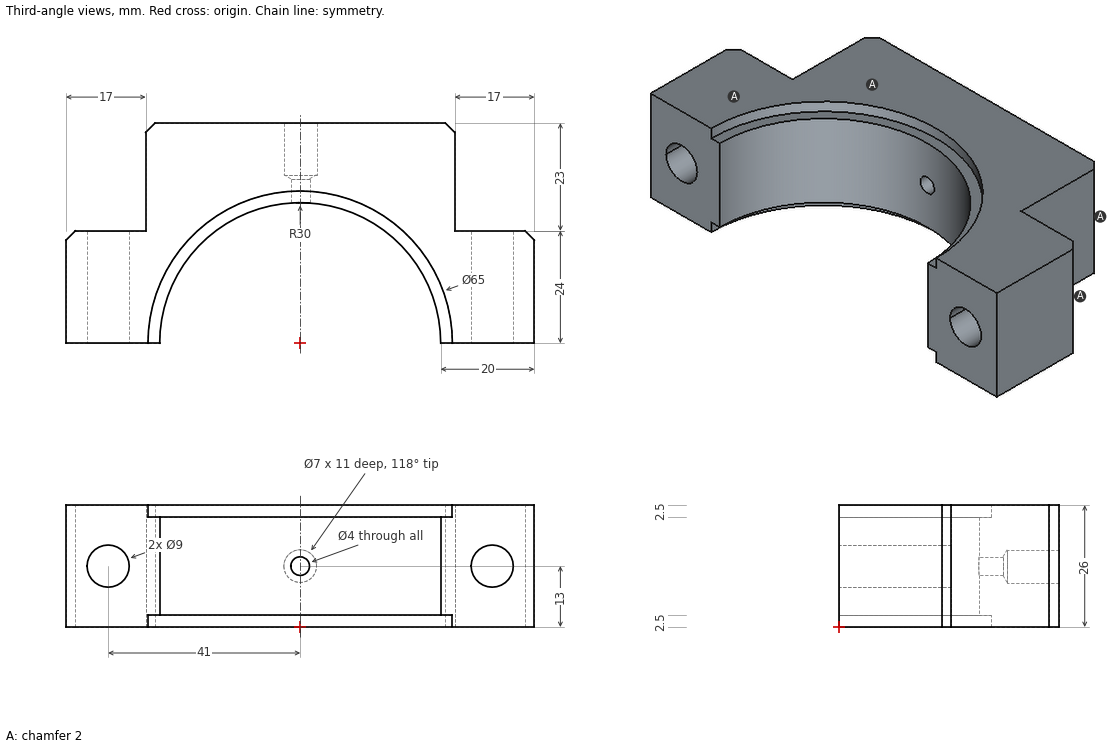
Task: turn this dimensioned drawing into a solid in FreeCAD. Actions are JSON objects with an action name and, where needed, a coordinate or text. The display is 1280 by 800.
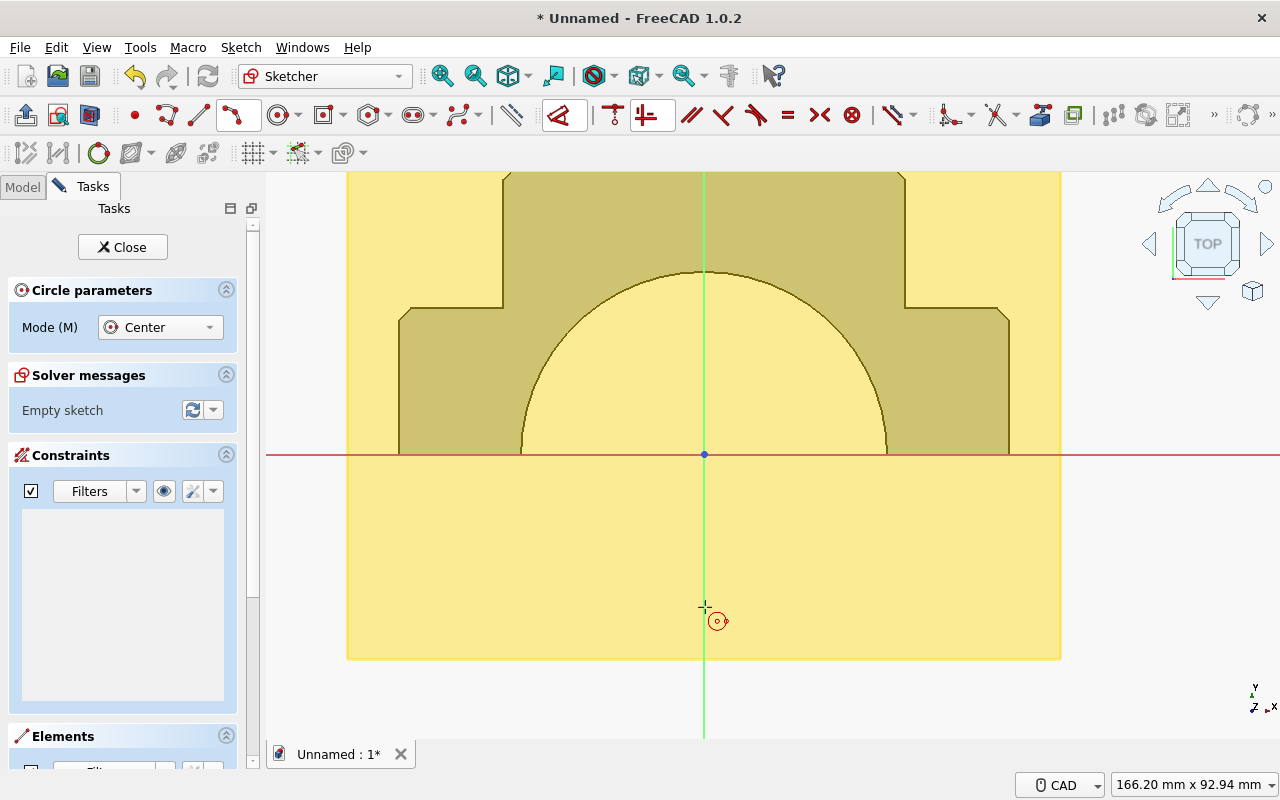
{"action": "left_click", "coordinate": [704, 455]}
{"action": "left_click", "coordinate": [844, 315]}
{"action": "key", "text": "Escape"}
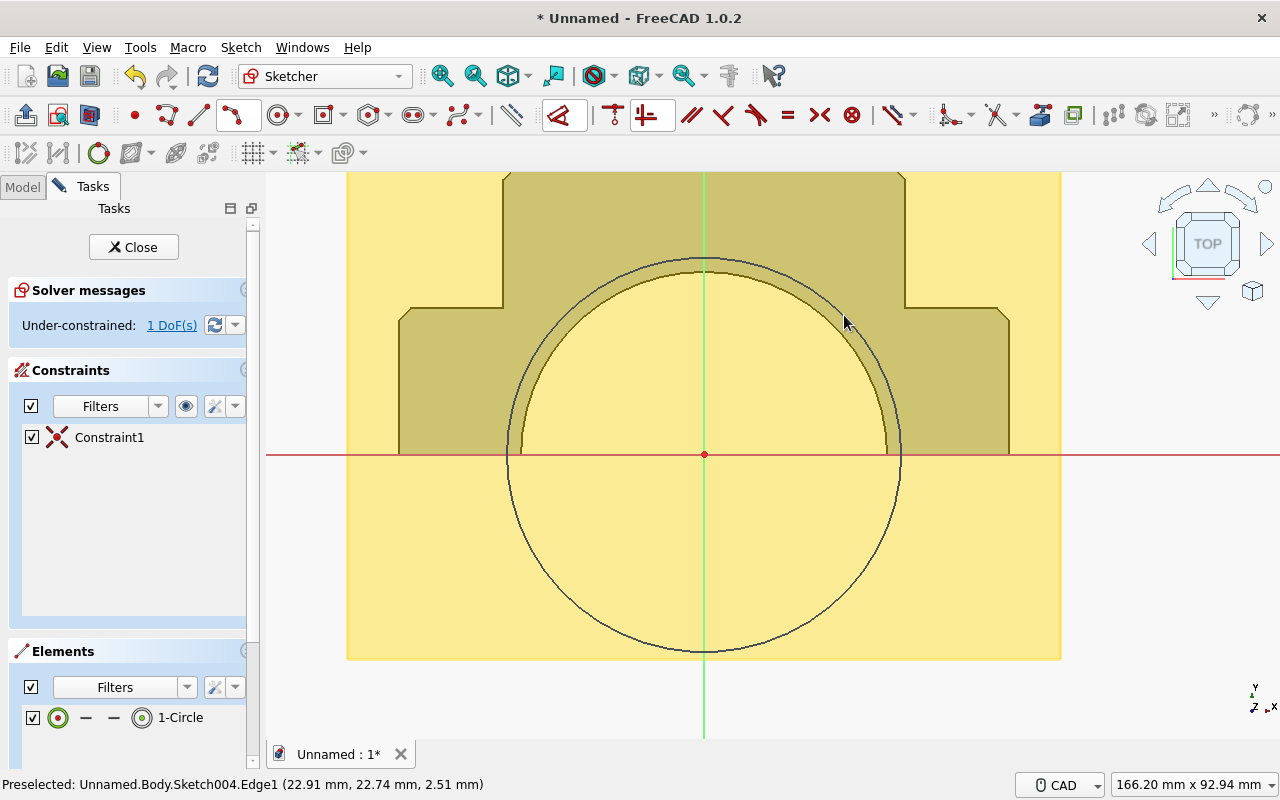
{"action": "left_click", "coordinate": [843, 315]}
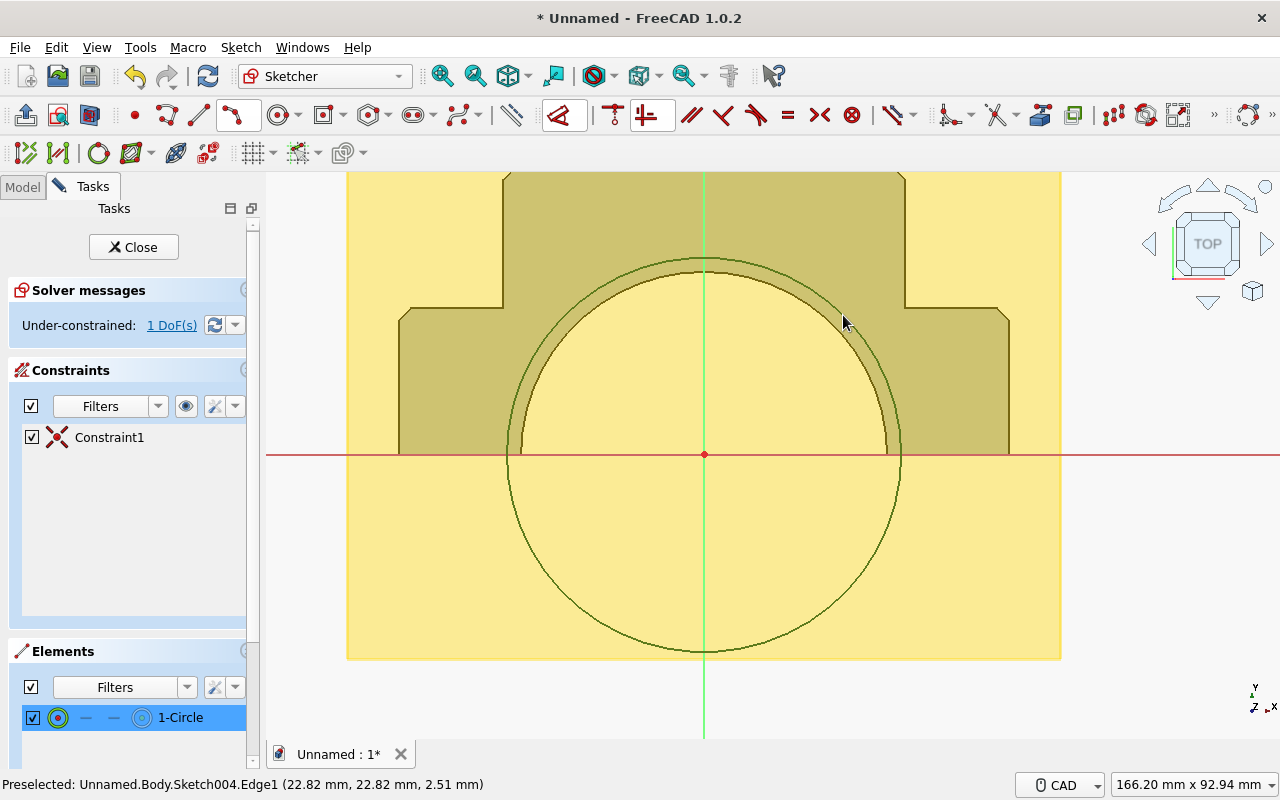
{"action": "key", "text": "k o"}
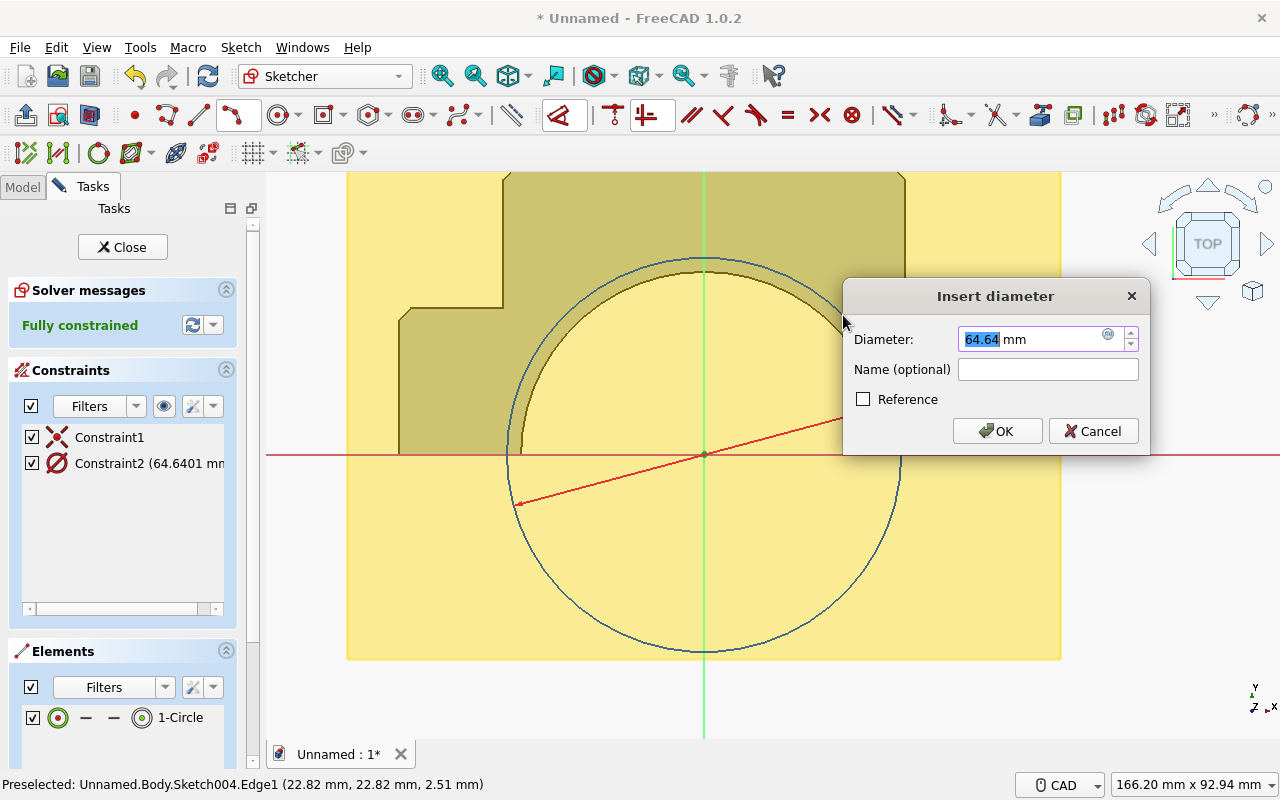
{"action": "type", "text": "65"}
{"action": "key", "text": "Return"}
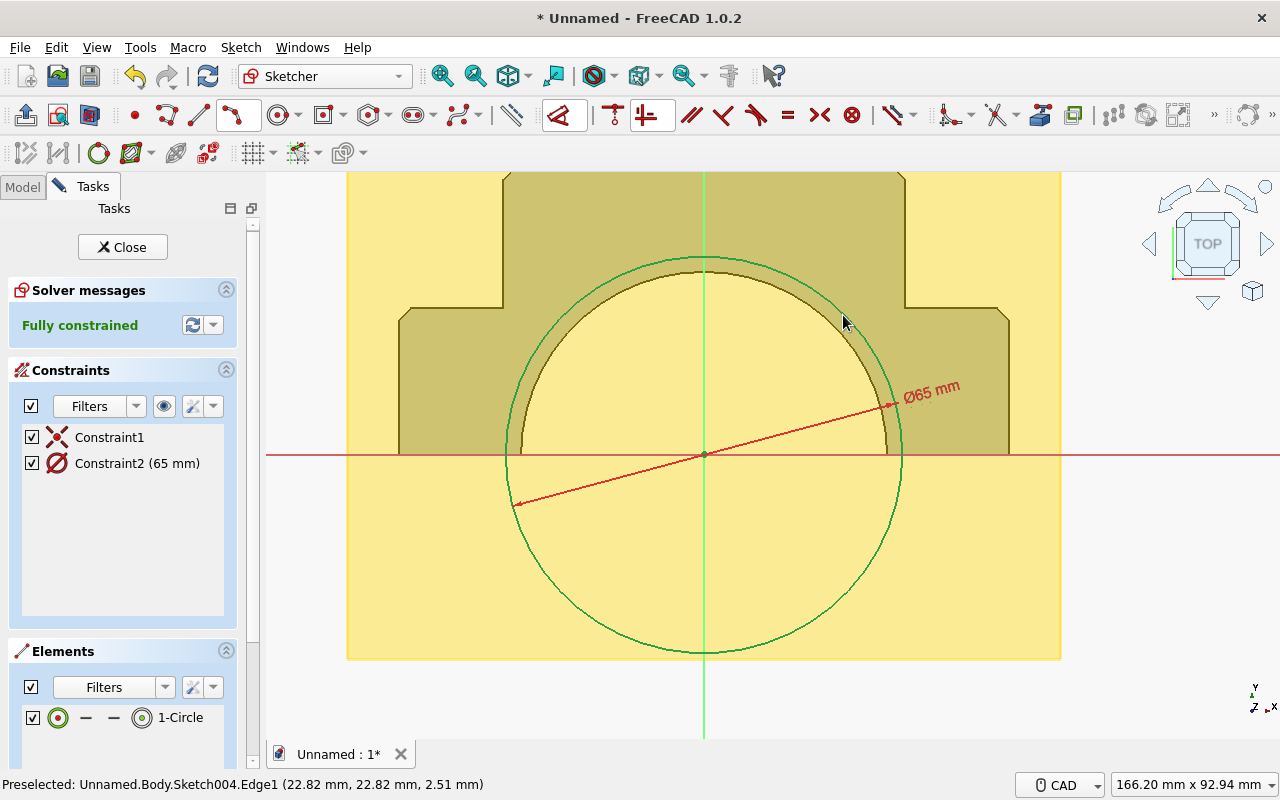
{"action": "left_click", "coordinate": [123, 247]}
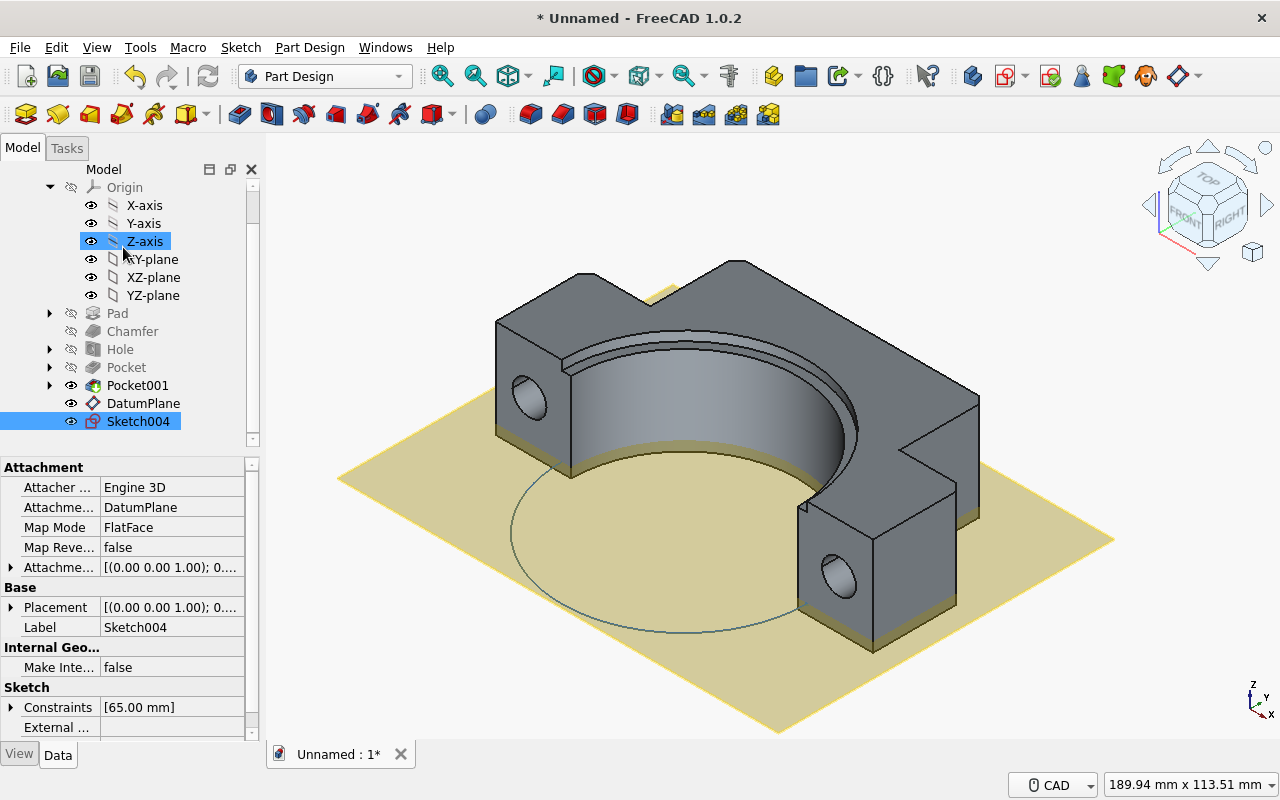
{"action": "left_click", "coordinate": [240, 114]}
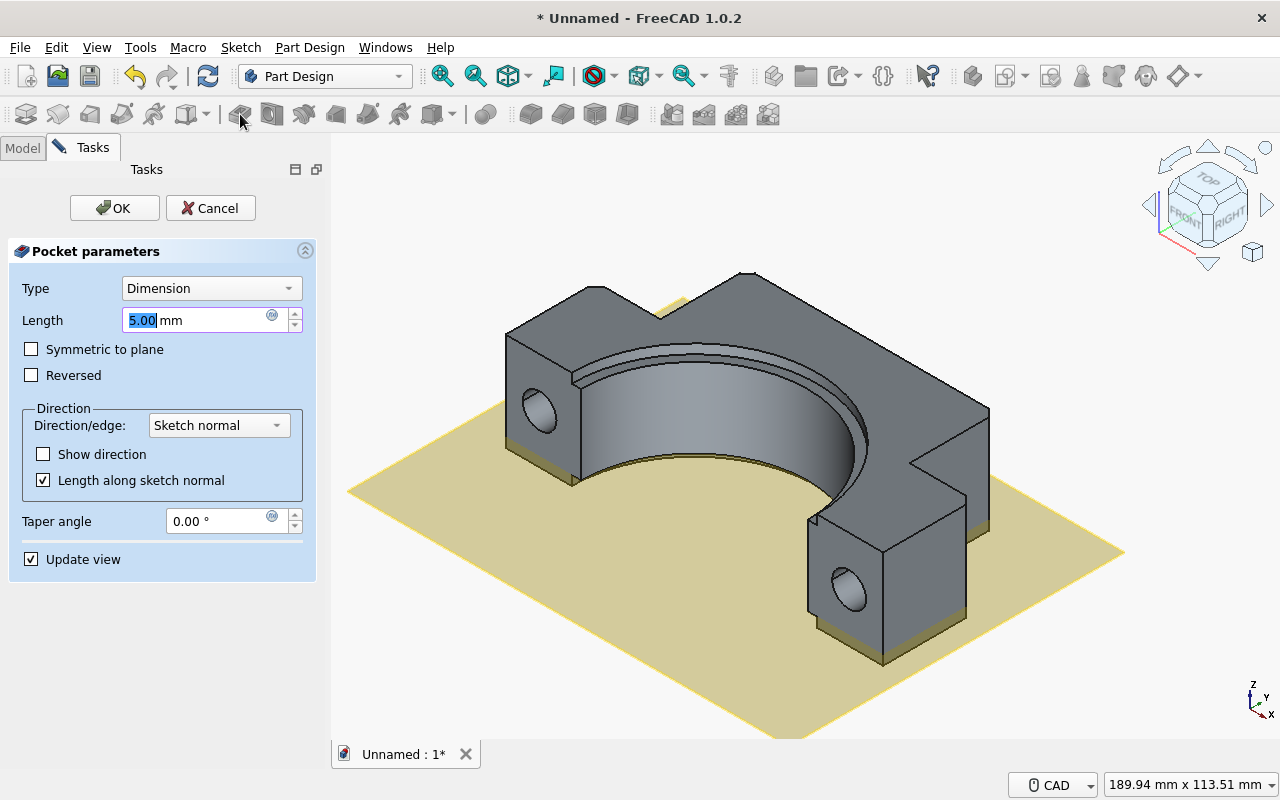
{"action": "type", "text": "2.5"}
{"action": "key", "text": "Tab"}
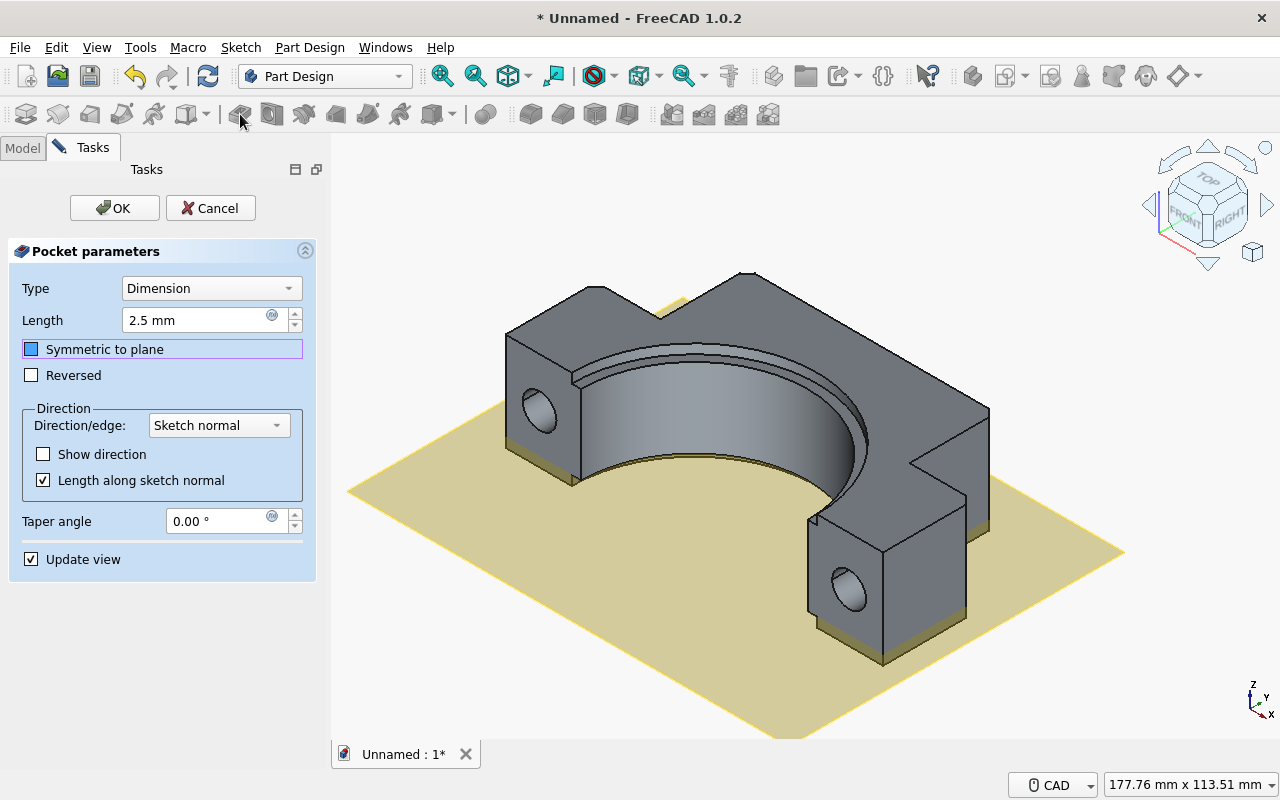
{"action": "left_click", "coordinate": [115, 208]}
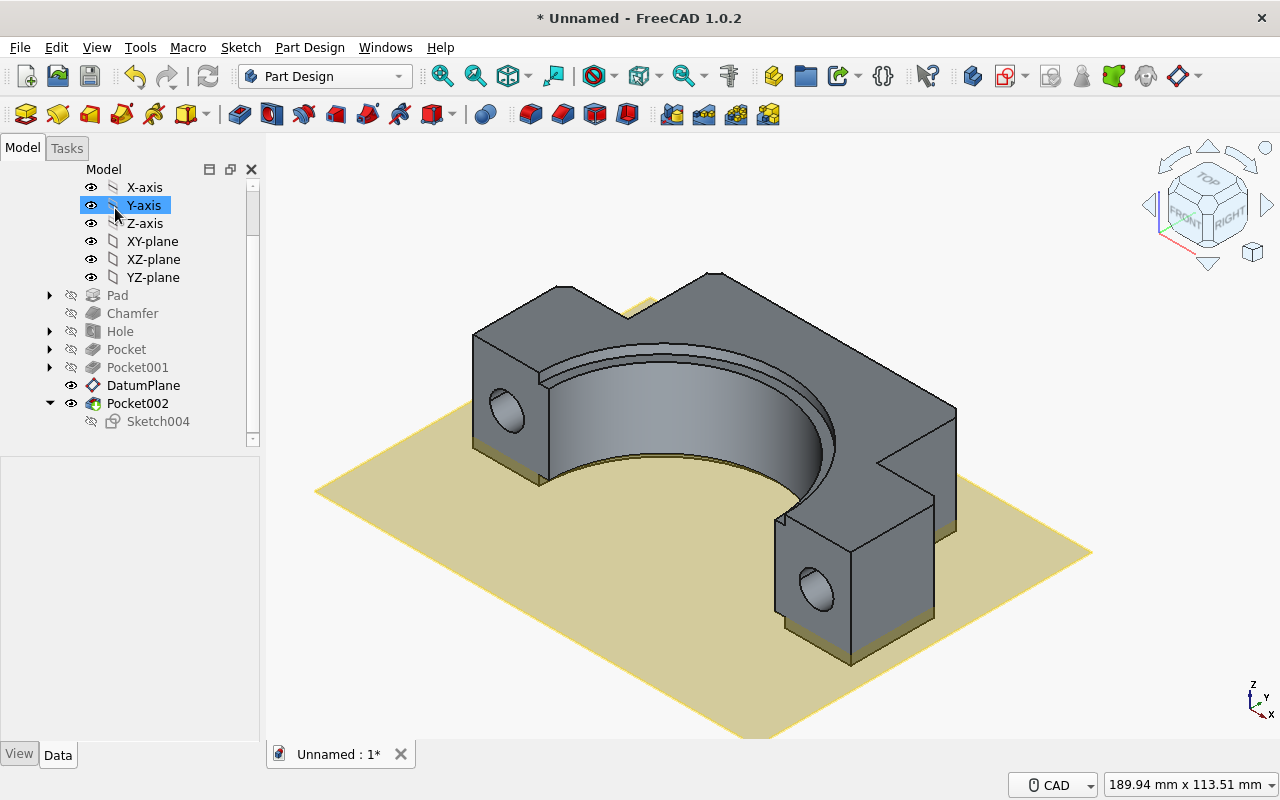
{"action": "left_click", "coordinate": [116, 385]}
{"action": "key", "text": "space"}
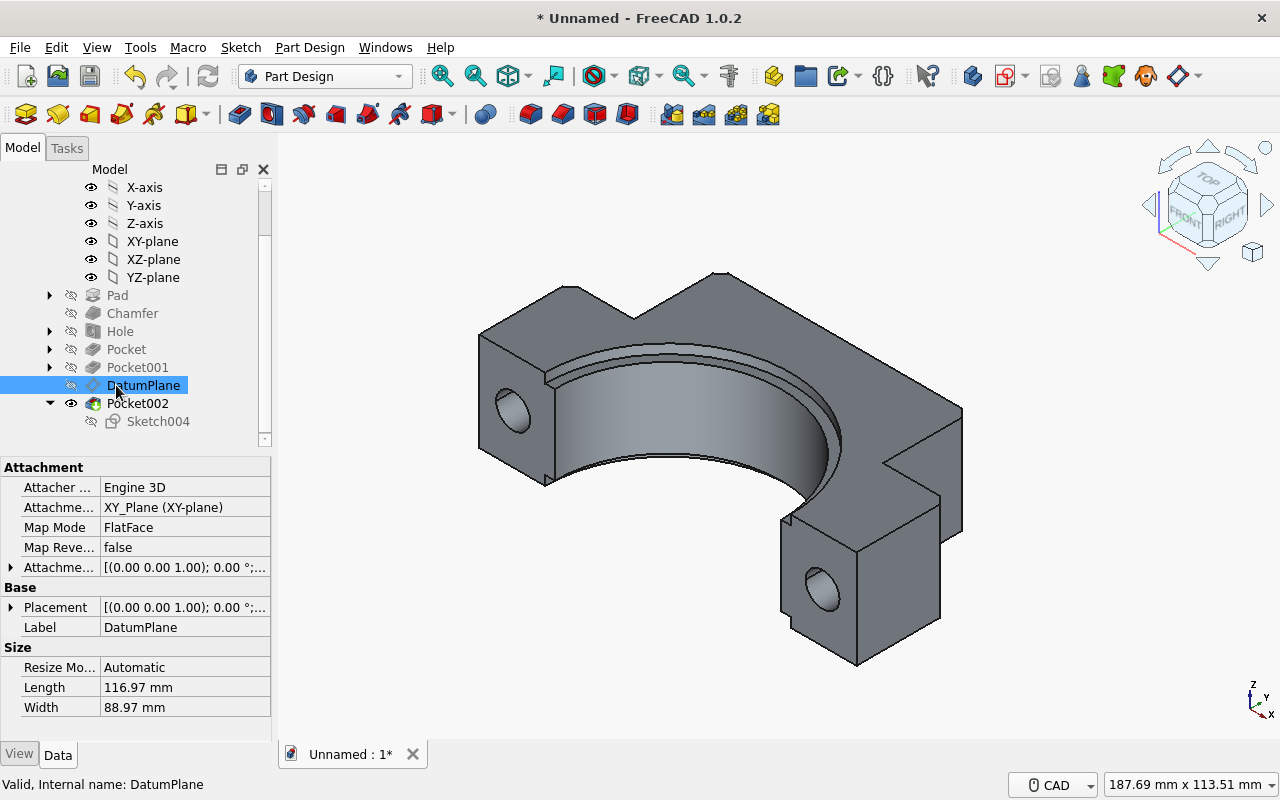
{"action": "key", "text": "4"}